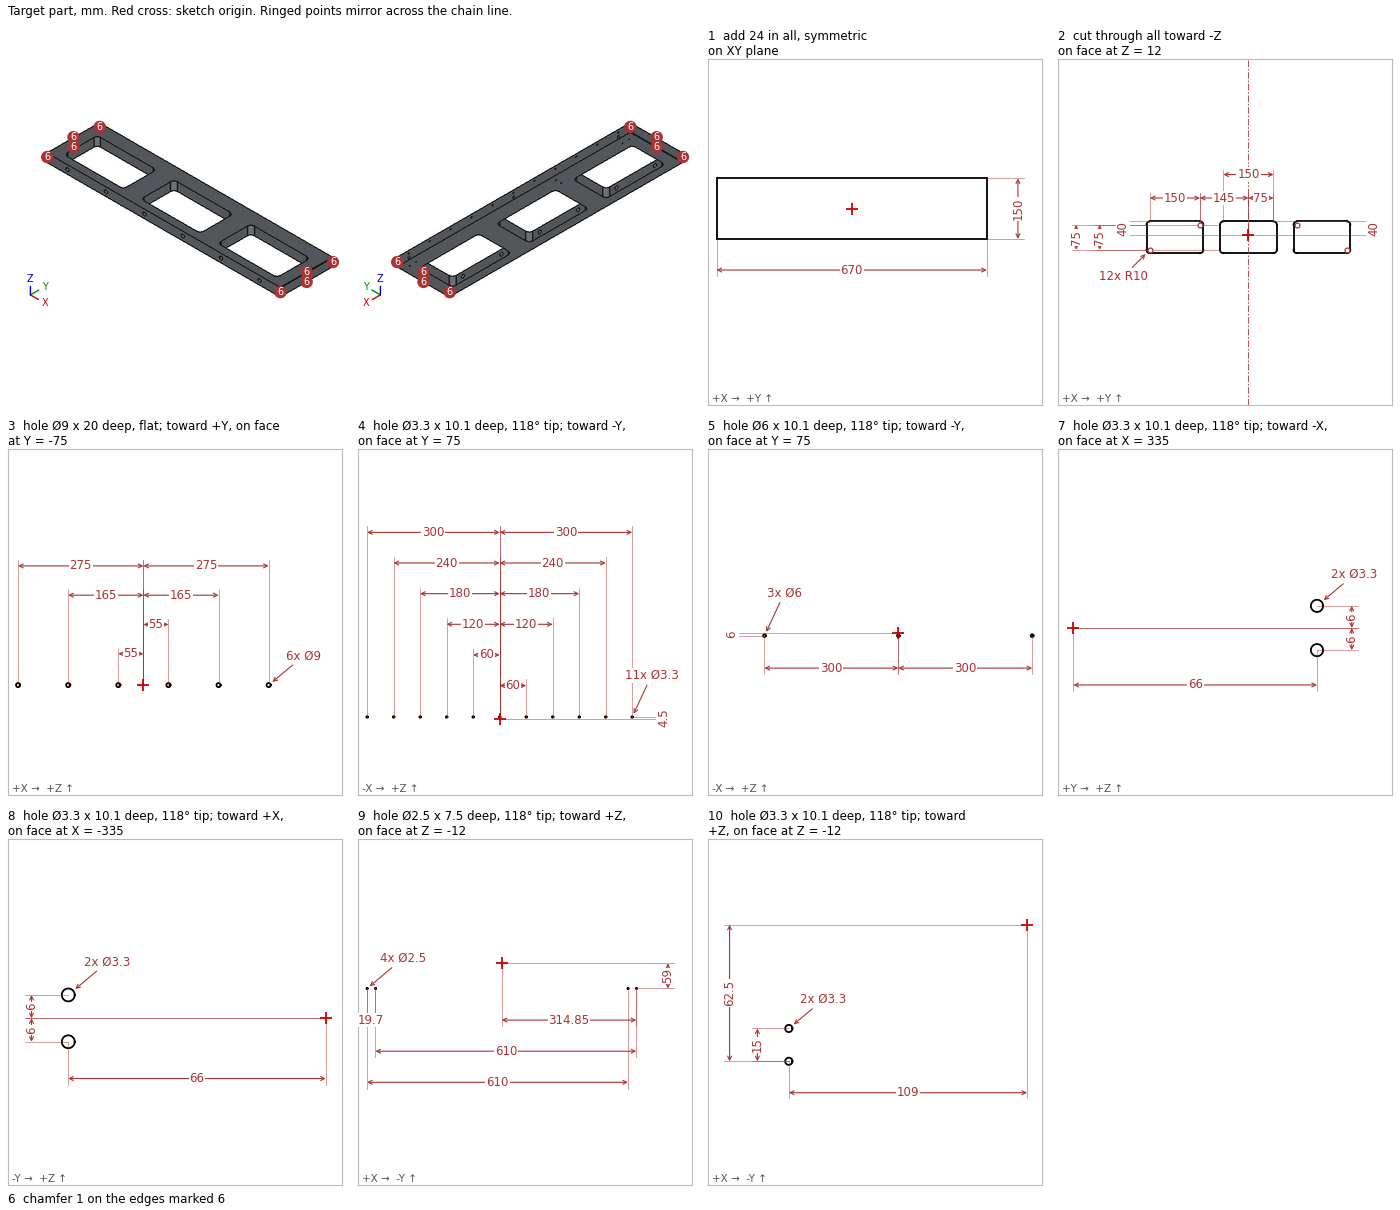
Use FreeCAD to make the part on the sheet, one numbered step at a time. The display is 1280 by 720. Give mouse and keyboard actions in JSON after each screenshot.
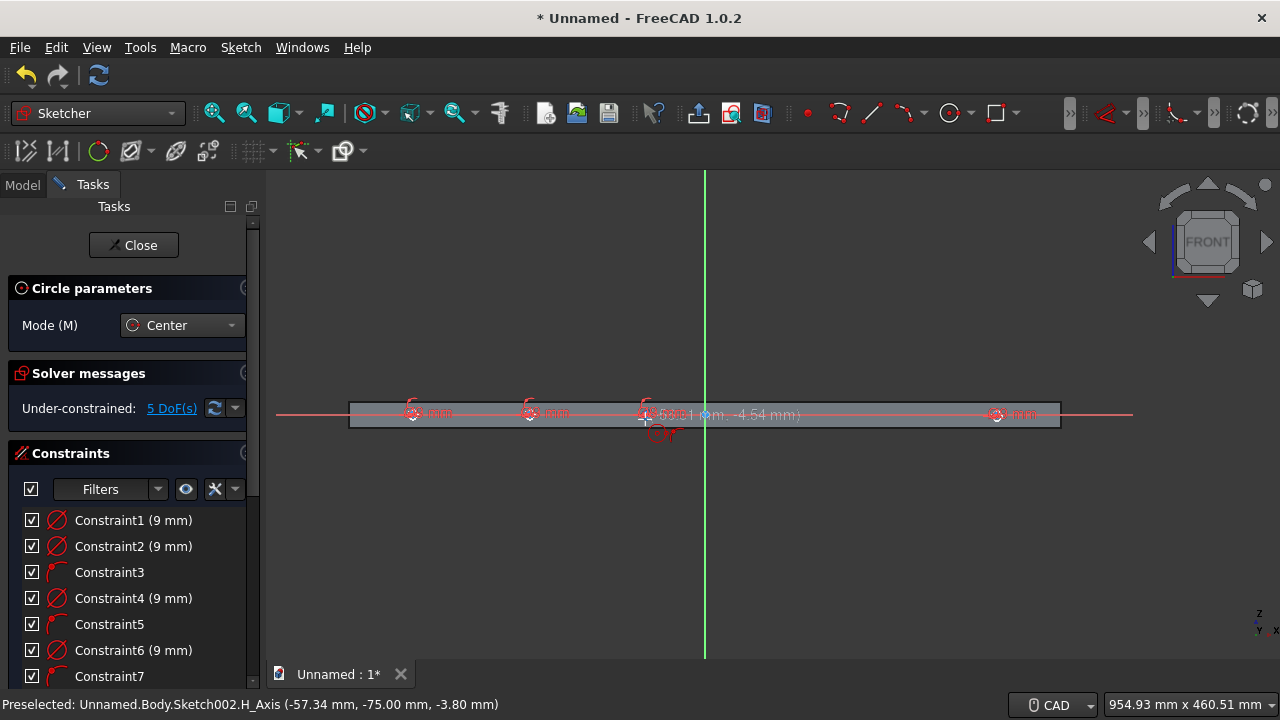
{"action": "scroll", "coordinate": [763, 415], "scroll_direction": "up", "scroll_amount": 8}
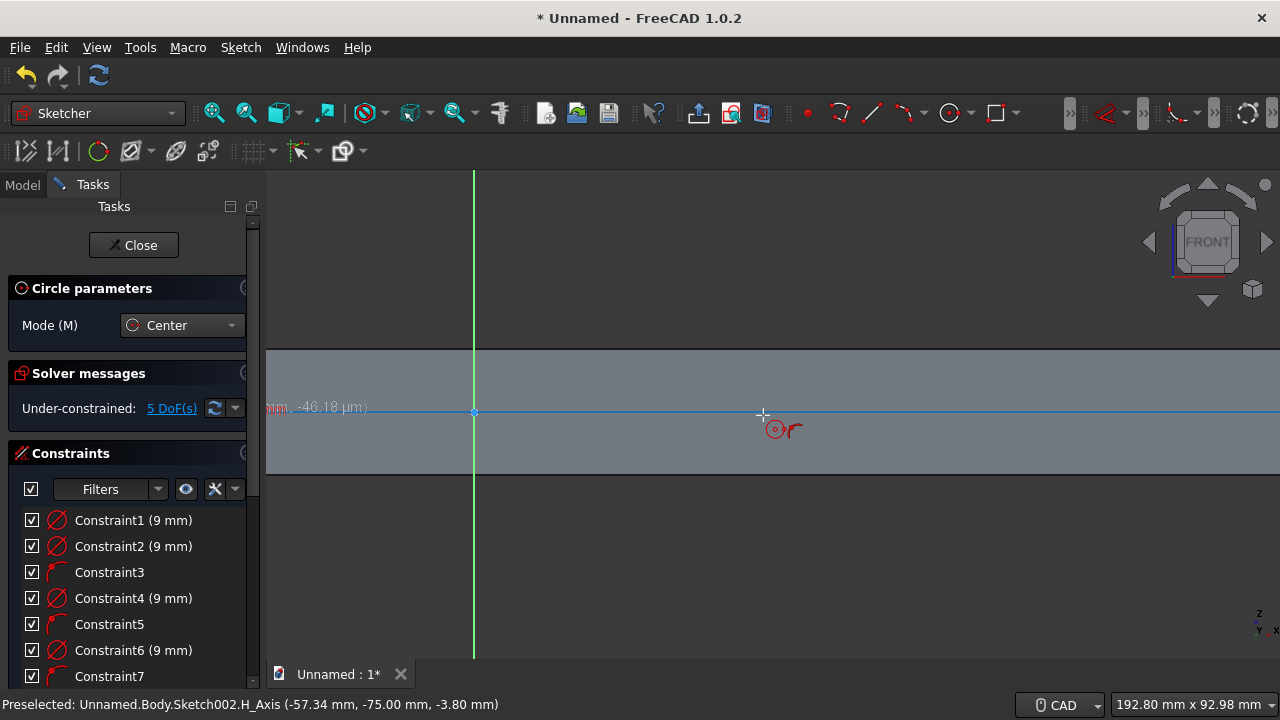
{"action": "scroll", "coordinate": [763, 415], "scroll_direction": "down", "scroll_amount": 8}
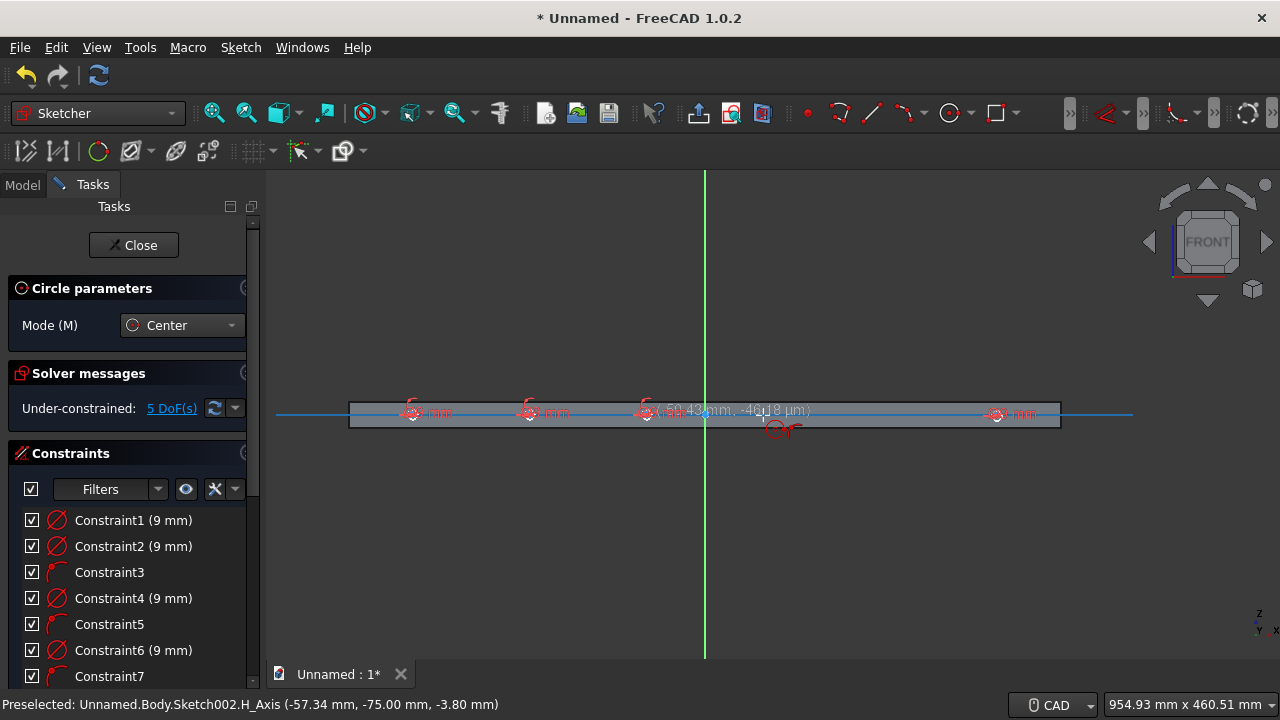
{"action": "left_click", "coordinate": [763, 415]}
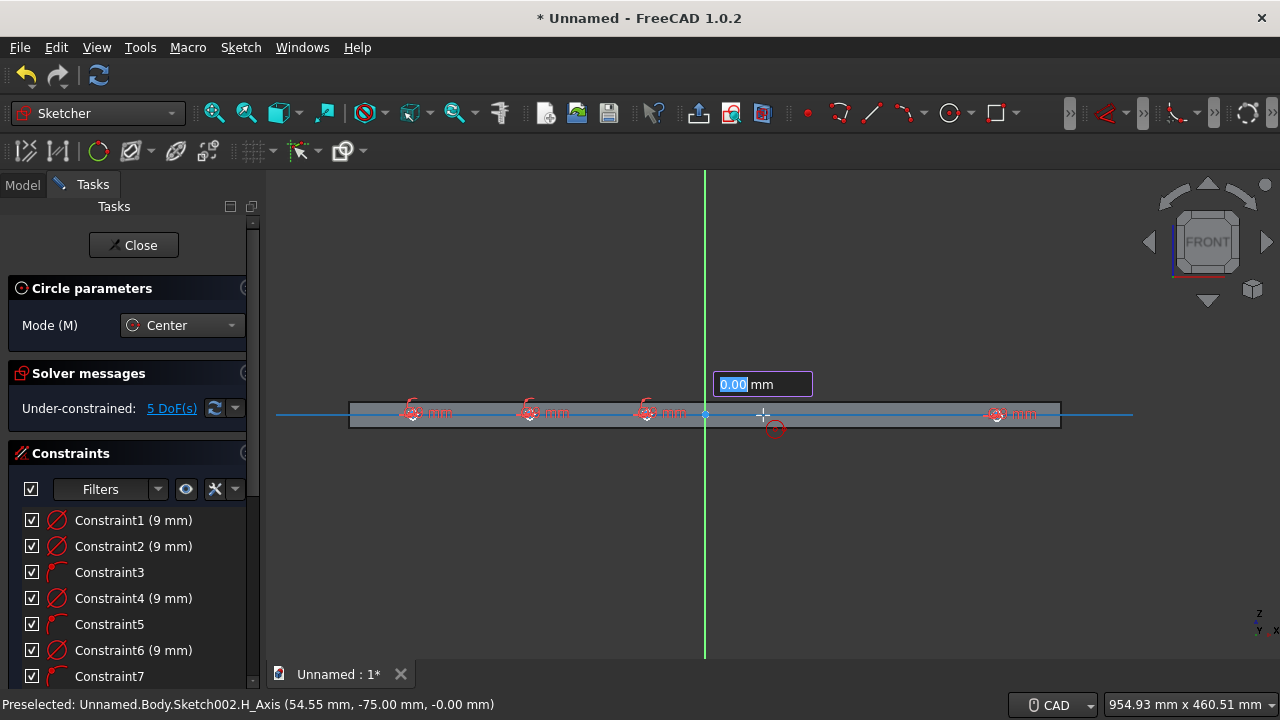
{"action": "scroll", "coordinate": [762, 419], "scroll_direction": "up", "scroll_amount": 7}
{"action": "mouse_move", "coordinate": [760, 419]}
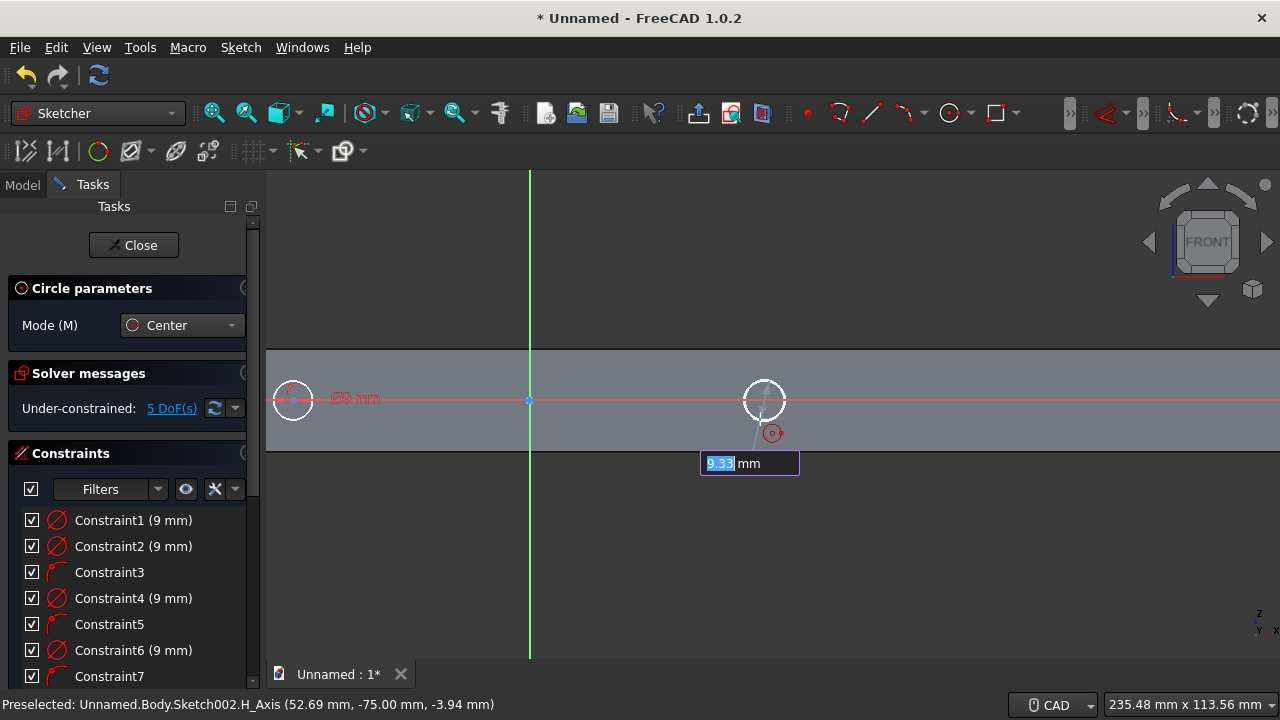
{"action": "type", "text": "9"}
{"action": "key", "text": "Return"}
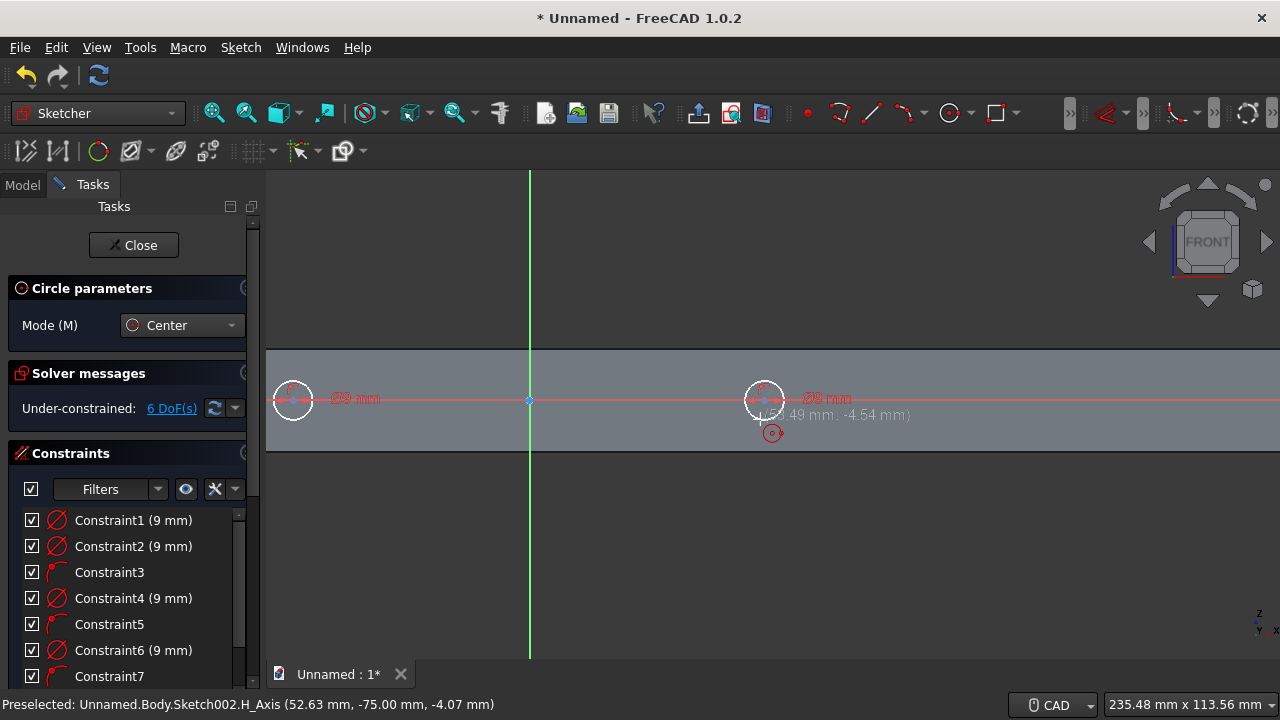
{"action": "scroll", "coordinate": [762, 419], "scroll_direction": "down", "scroll_amount": 7}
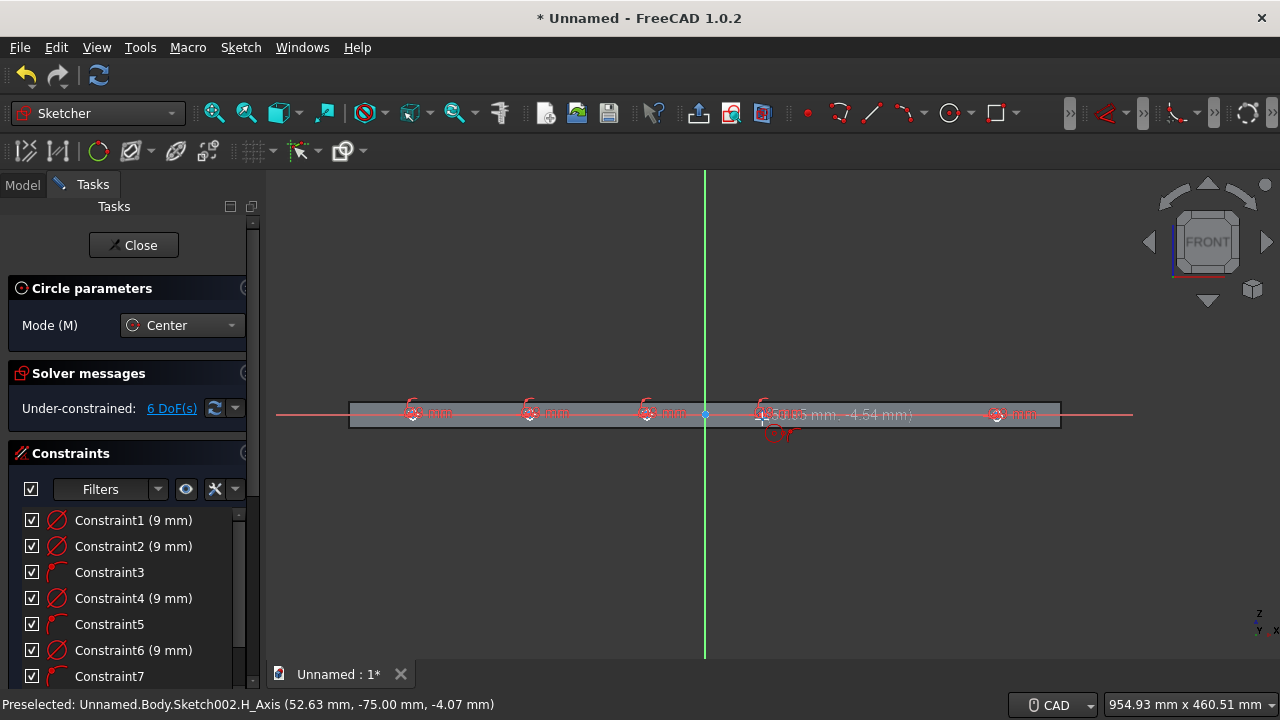
{"action": "scroll", "coordinate": [880, 415], "scroll_direction": "up", "scroll_amount": 8}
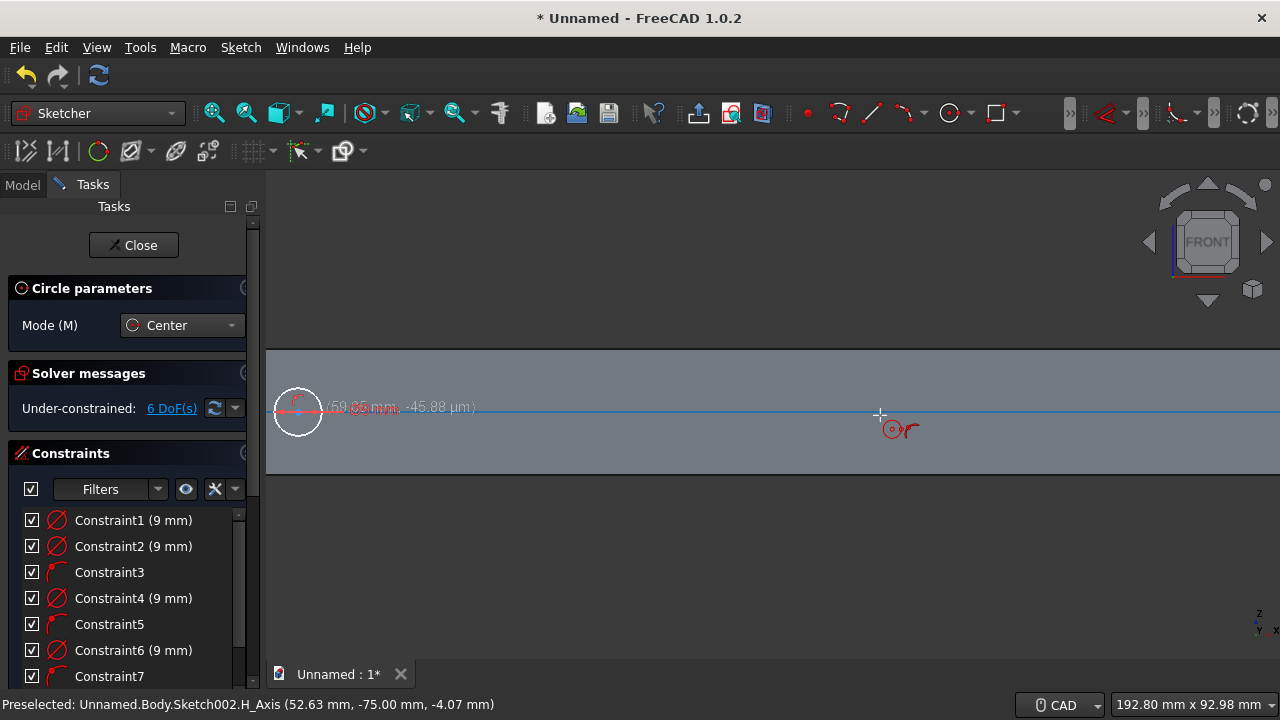
{"action": "scroll", "coordinate": [880, 415], "scroll_direction": "down", "scroll_amount": 8}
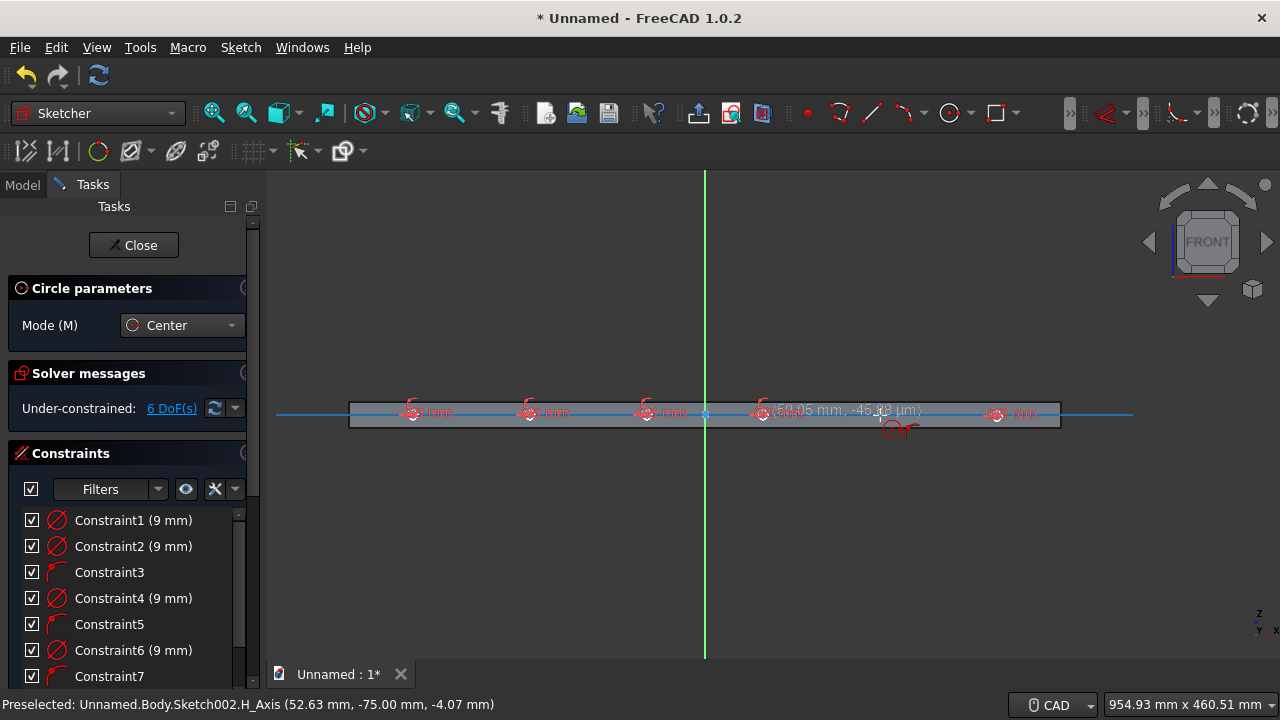
{"action": "left_click", "coordinate": [880, 415]}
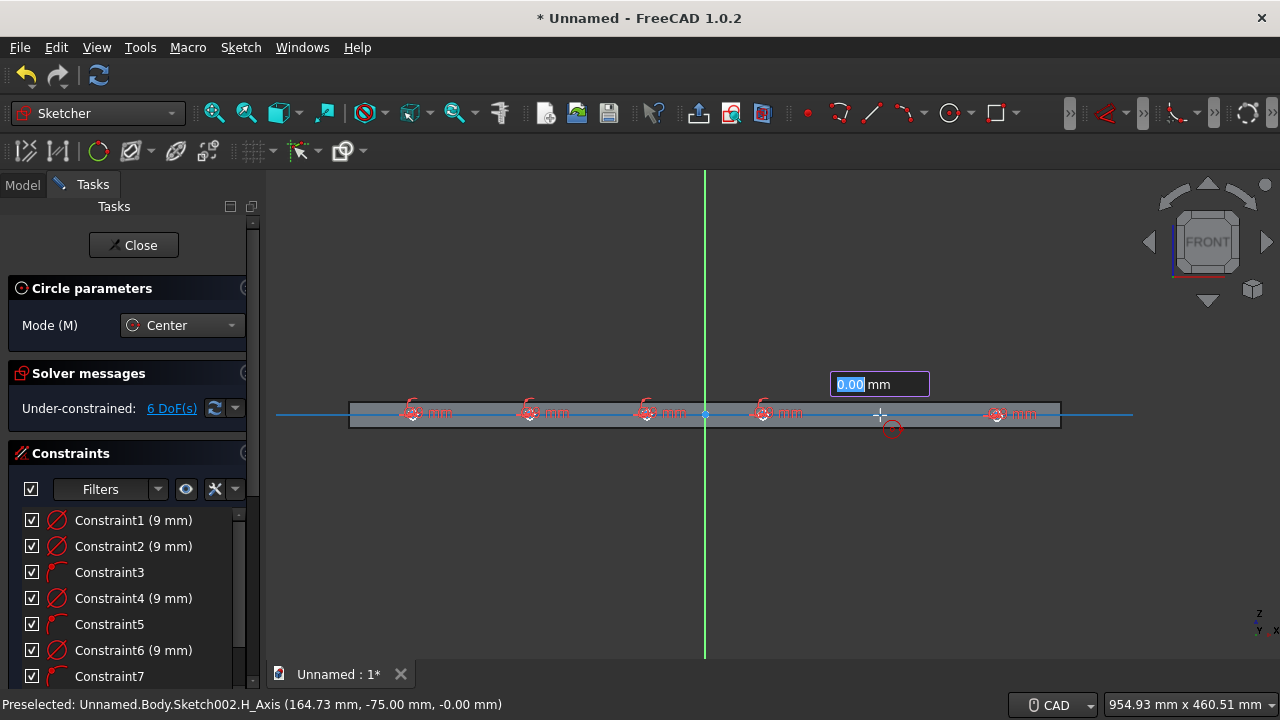
{"action": "scroll", "coordinate": [879, 419], "scroll_direction": "up", "scroll_amount": 7}
{"action": "mouse_move", "coordinate": [876, 419]}